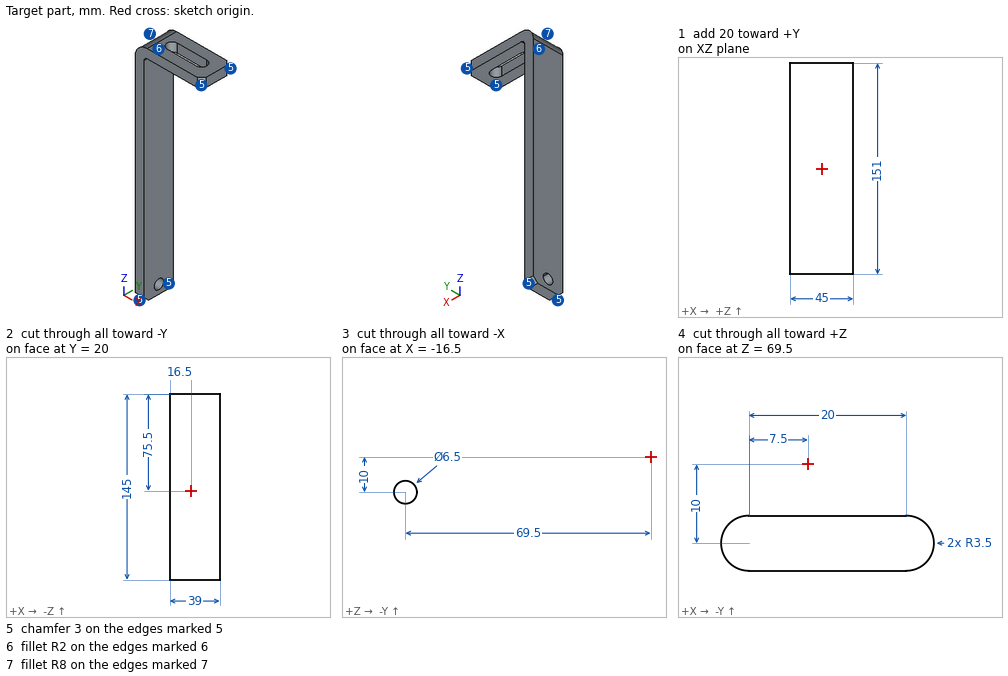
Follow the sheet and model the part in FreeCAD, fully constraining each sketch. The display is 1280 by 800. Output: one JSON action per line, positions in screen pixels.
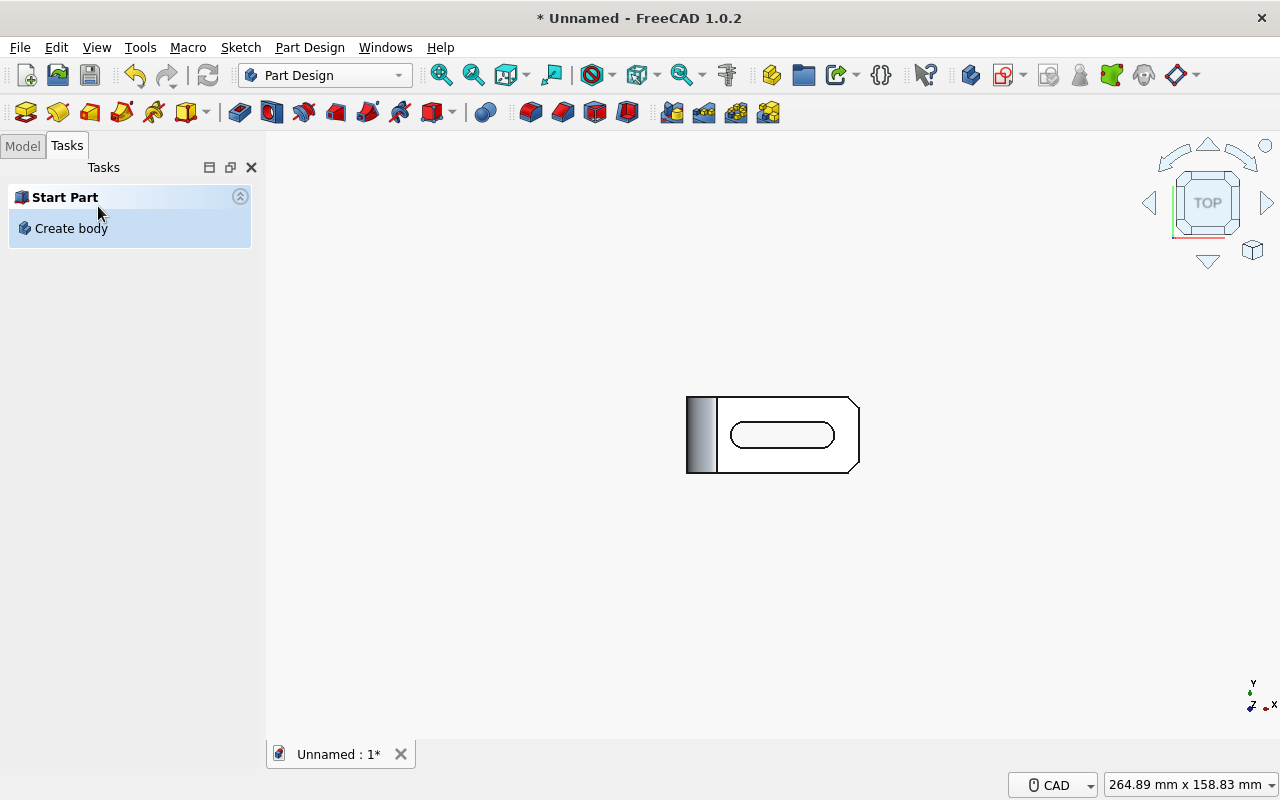
{"action": "key", "text": "0"}